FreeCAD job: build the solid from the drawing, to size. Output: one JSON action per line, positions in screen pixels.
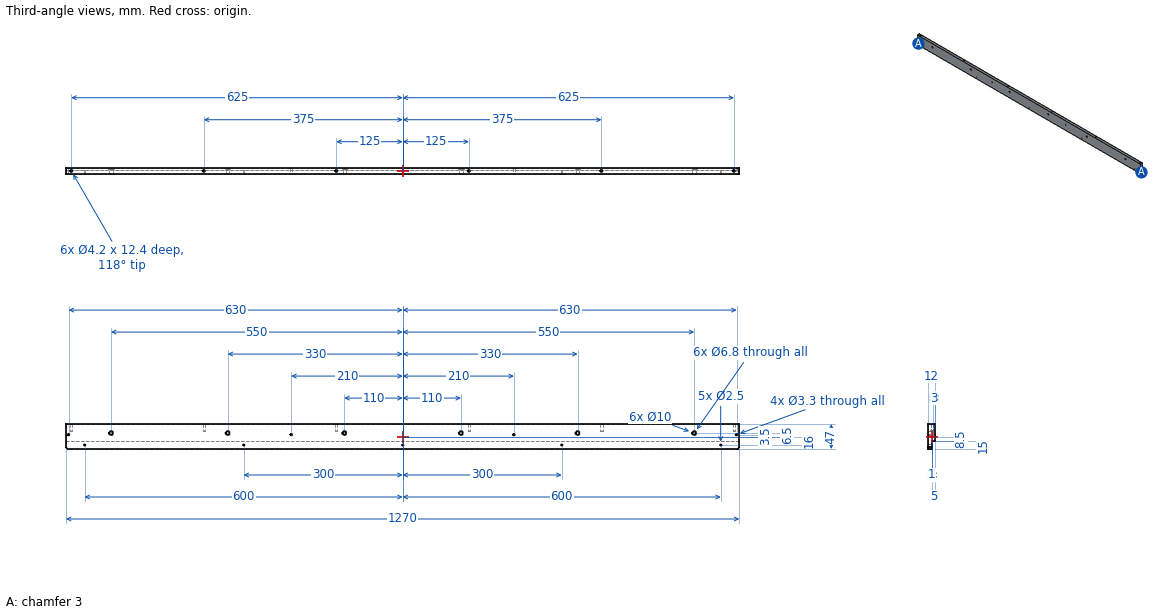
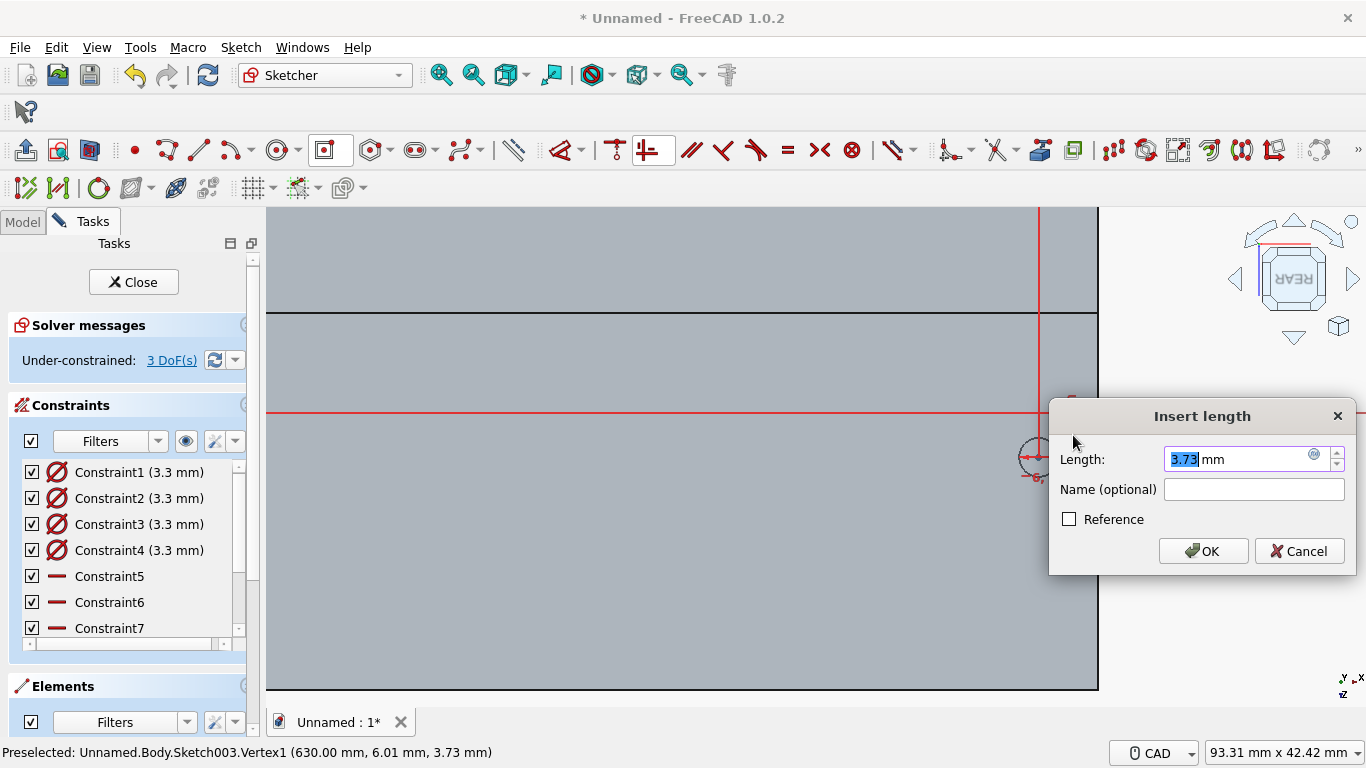
{"action": "type", "text": "3.5"}
{"action": "key", "text": "Return"}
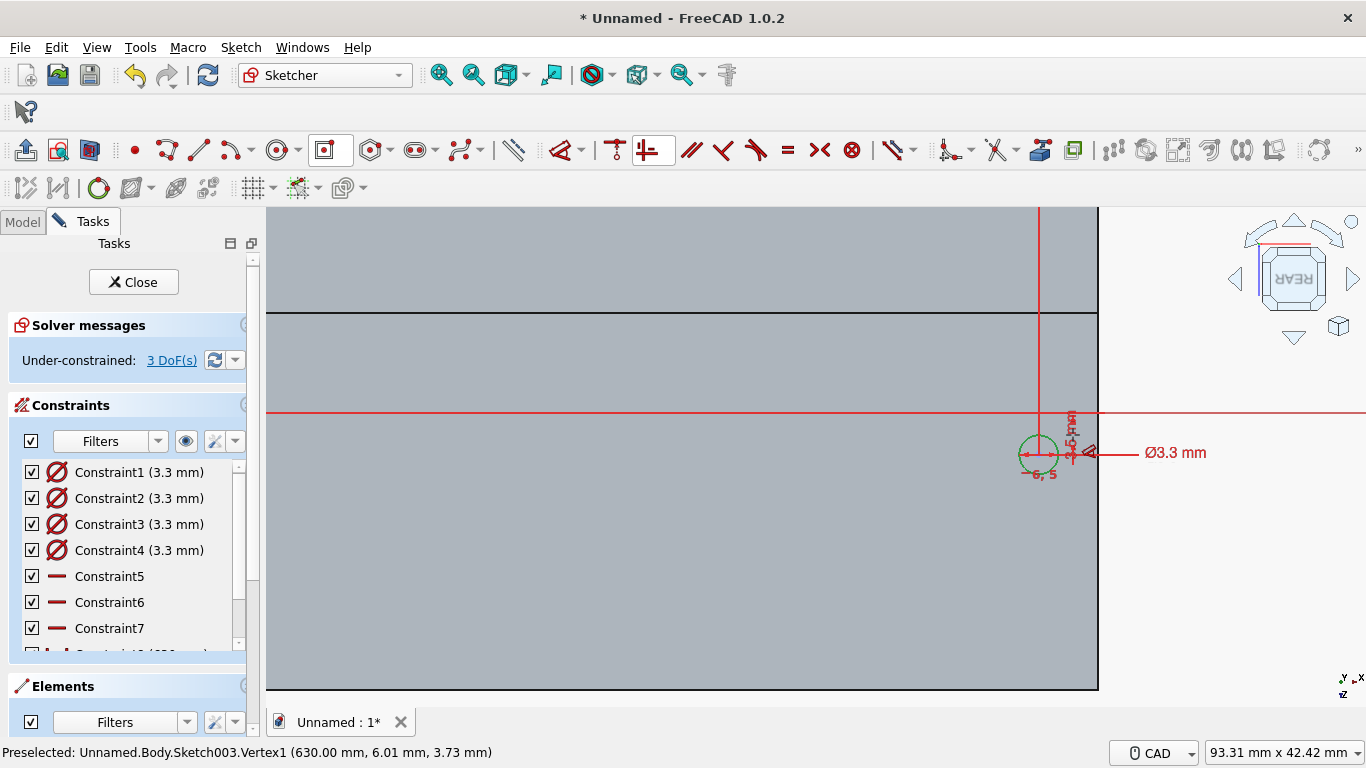
{"action": "scroll", "coordinate": [1121, 458], "scroll_direction": "down", "scroll_amount": 15}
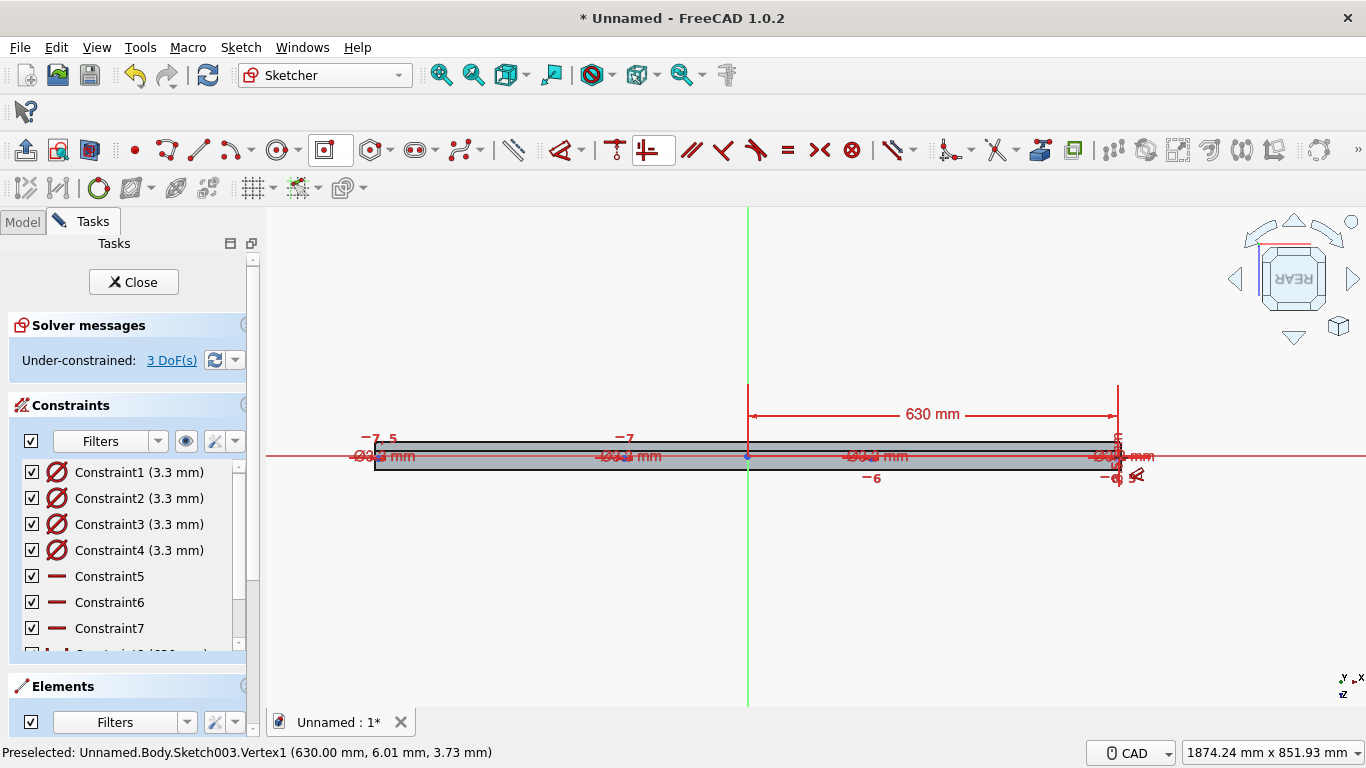
{"action": "left_click", "coordinate": [378, 458]}
{"action": "left_click", "coordinate": [563, 422]}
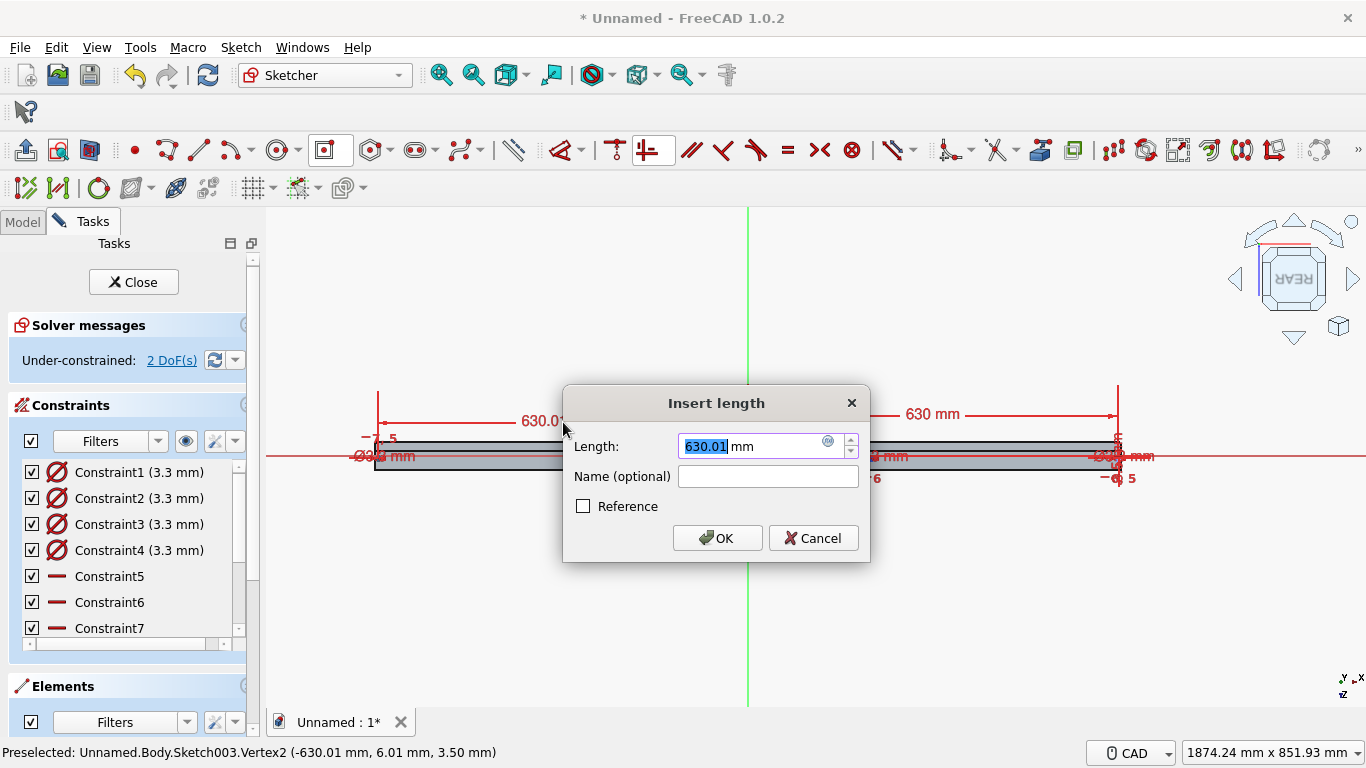
{"action": "type", "text": "630"}
{"action": "key", "text": "Return"}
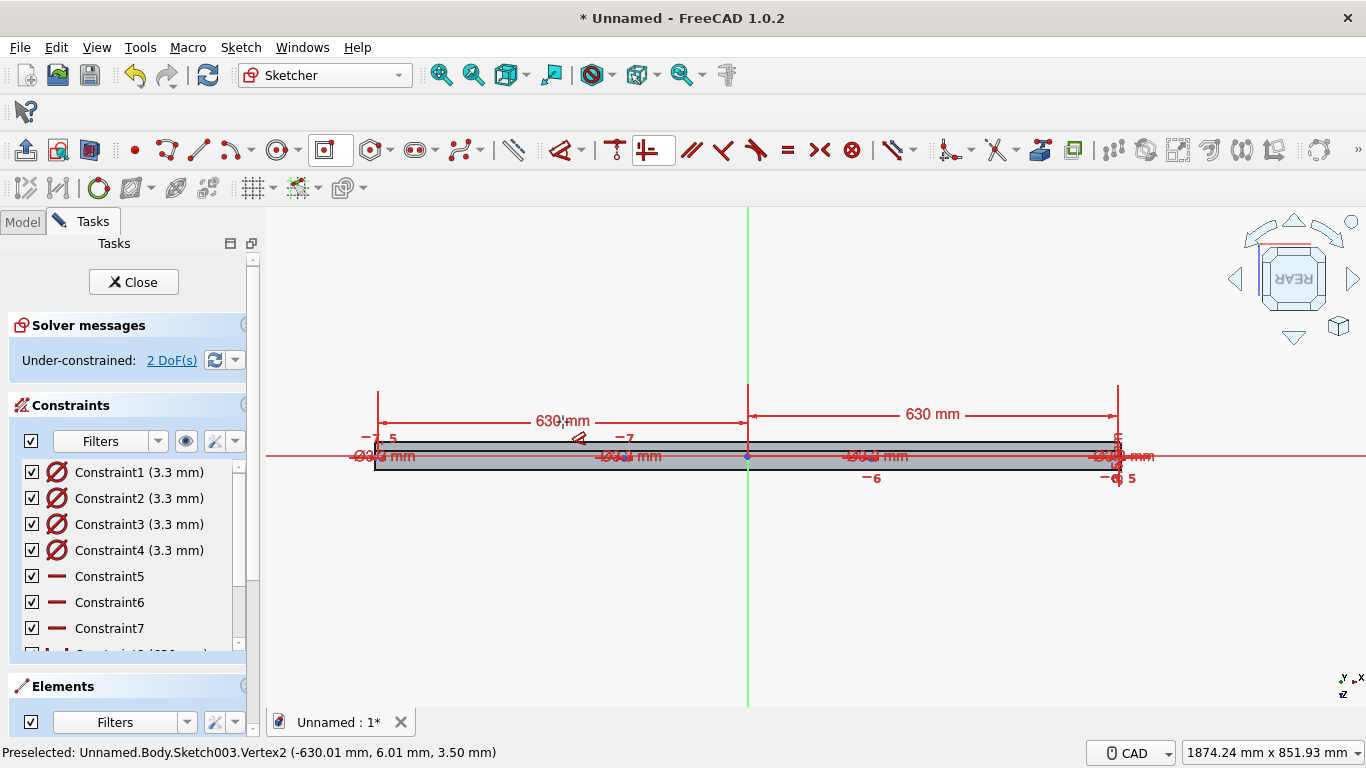
{"action": "left_click", "coordinate": [871, 458]}
{"action": "left_click", "coordinate": [810, 422]}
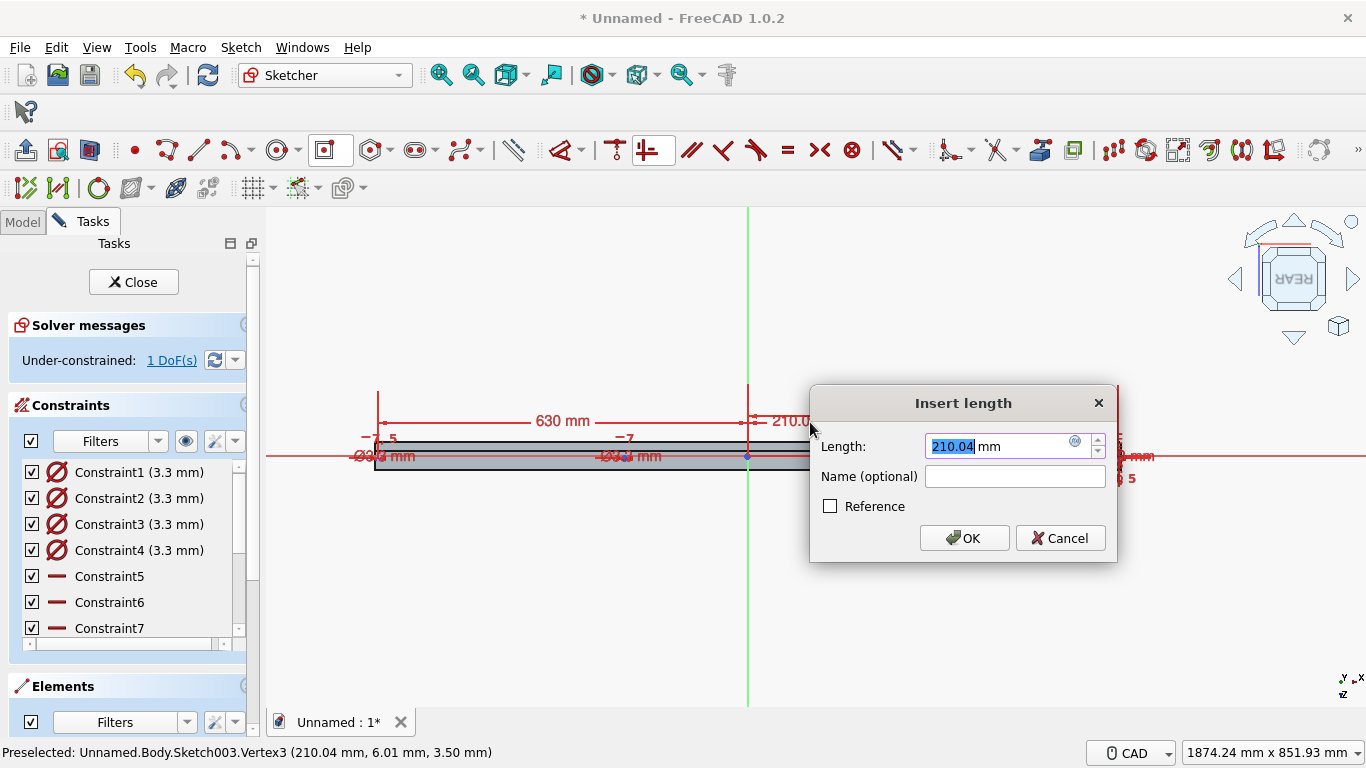
{"action": "type", "text": "210"}
{"action": "key", "text": "Return"}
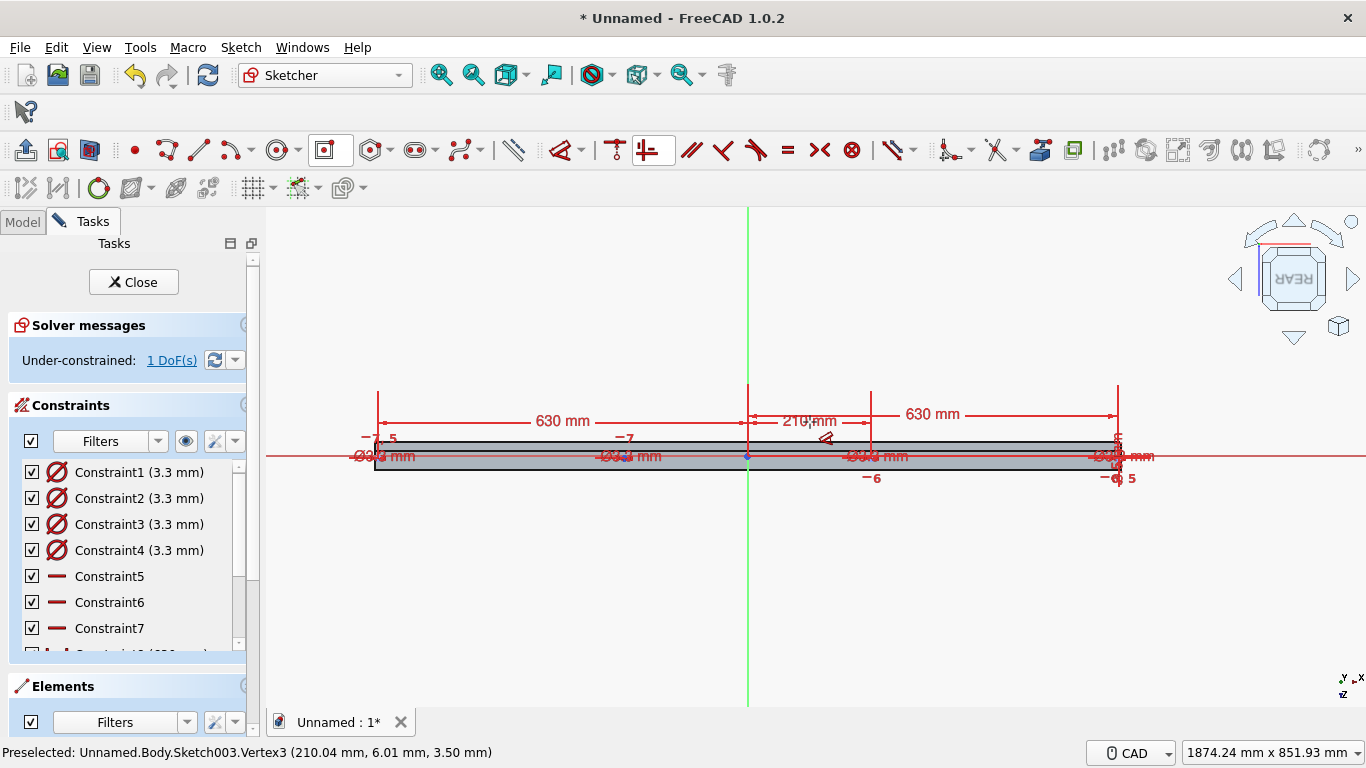
{"action": "left_click", "coordinate": [625, 458]}
{"action": "left_click", "coordinate": [686, 422]}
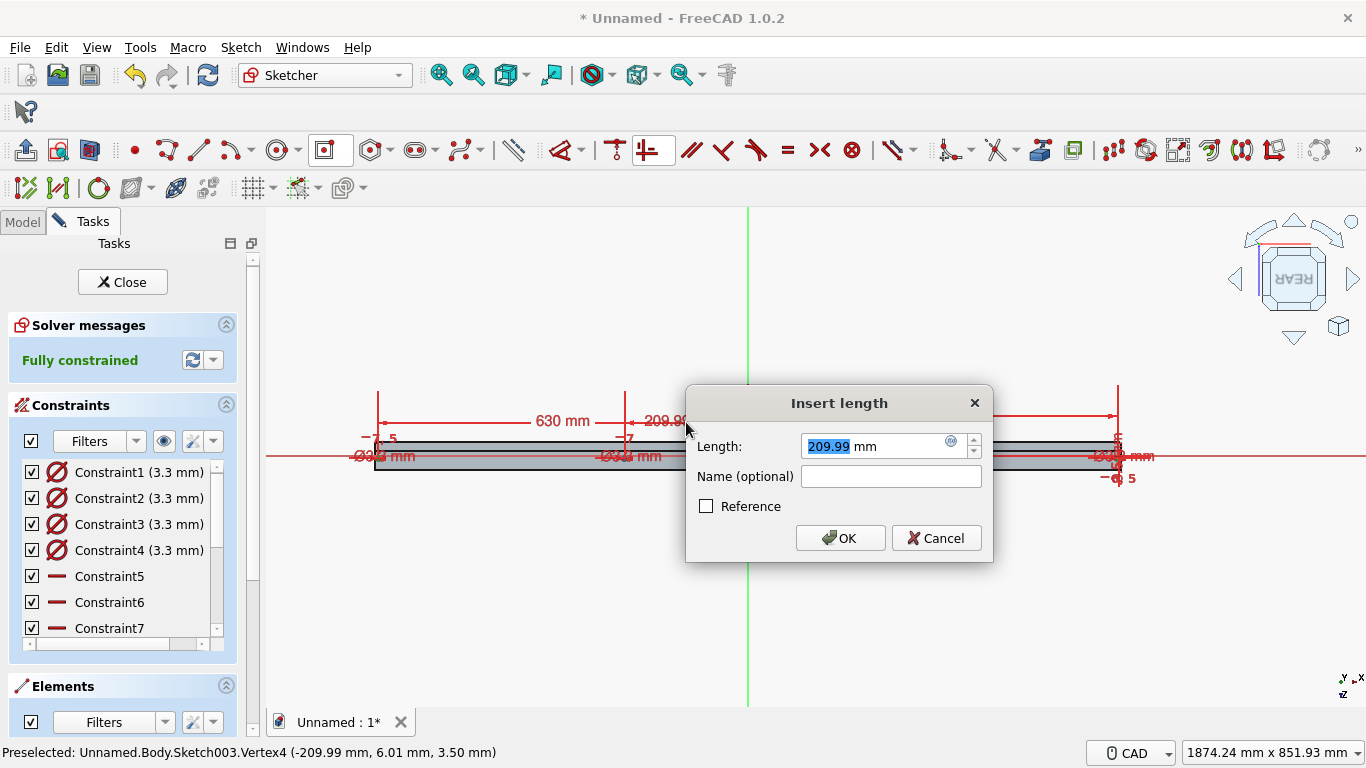
{"action": "type", "text": "210"}
{"action": "key", "text": "Return"}
{"action": "key", "text": "Escape"}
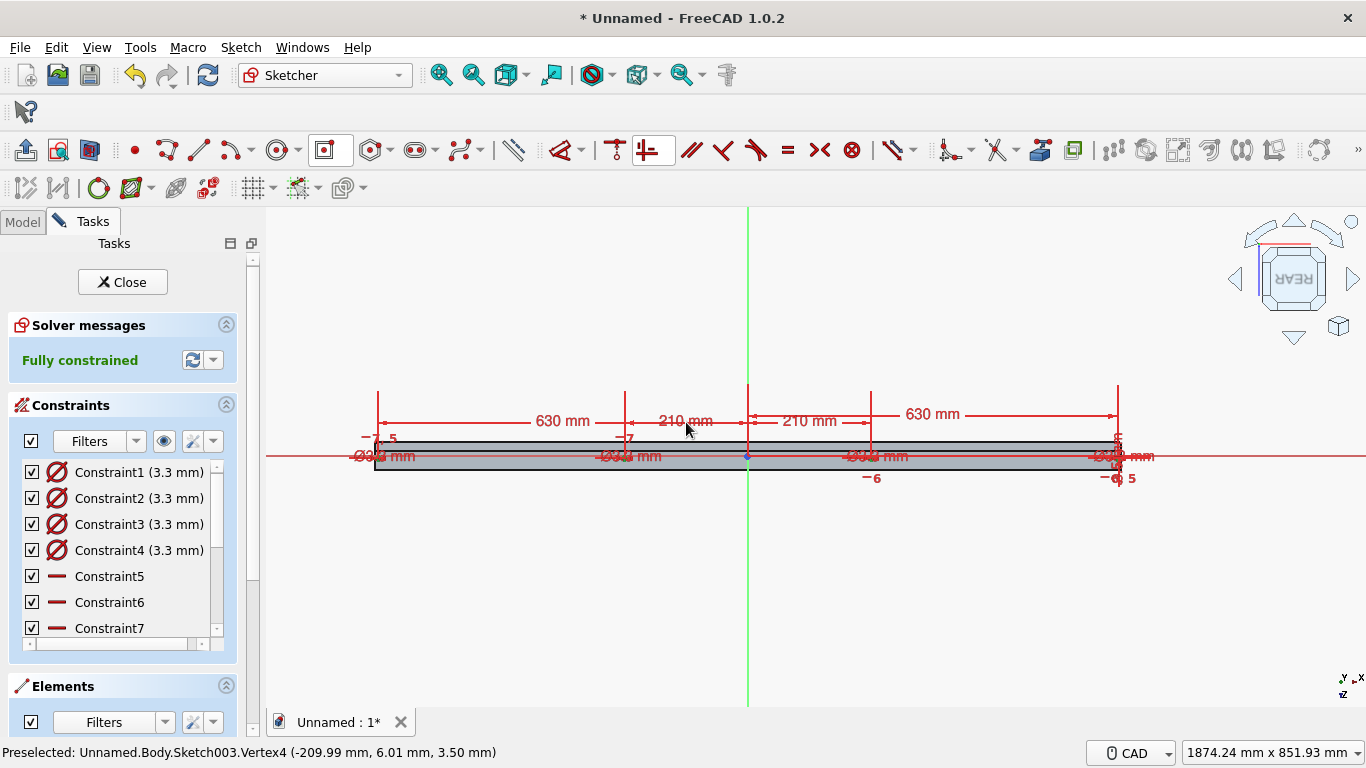
{"action": "left_click", "coordinate": [123, 282]}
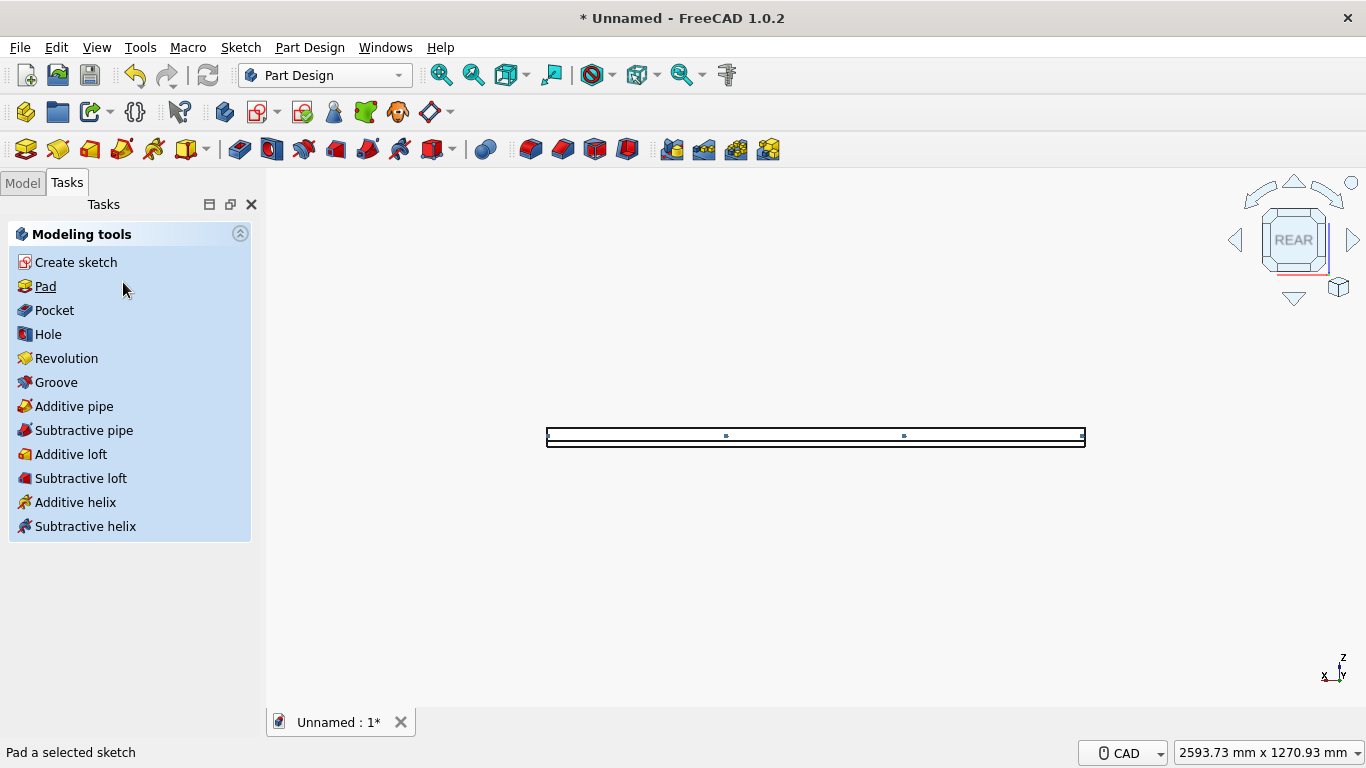
{"action": "left_click", "coordinate": [272, 150]}